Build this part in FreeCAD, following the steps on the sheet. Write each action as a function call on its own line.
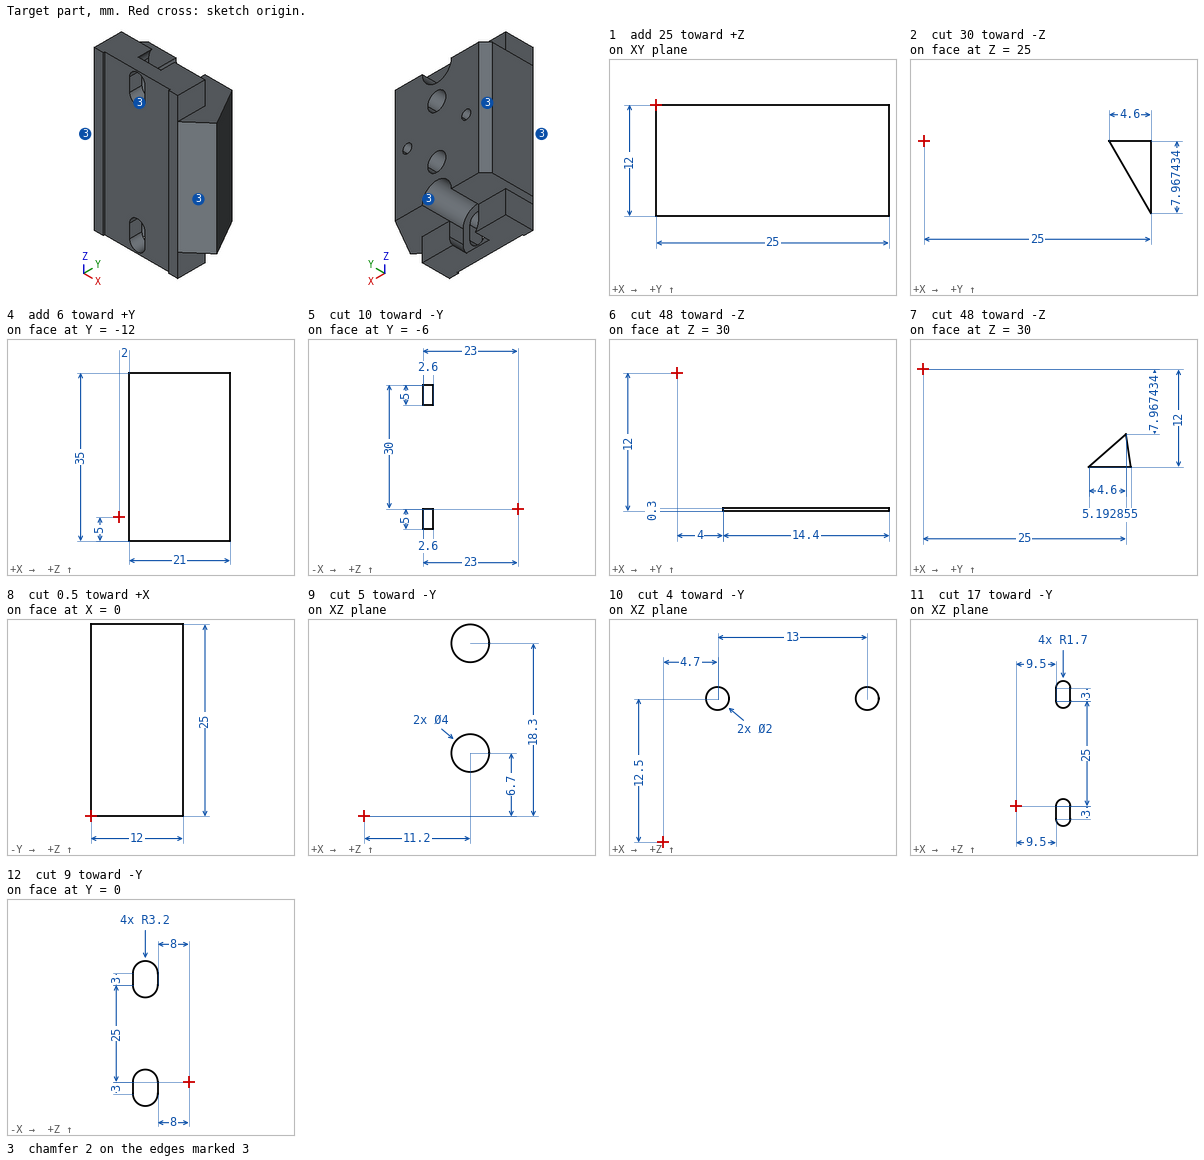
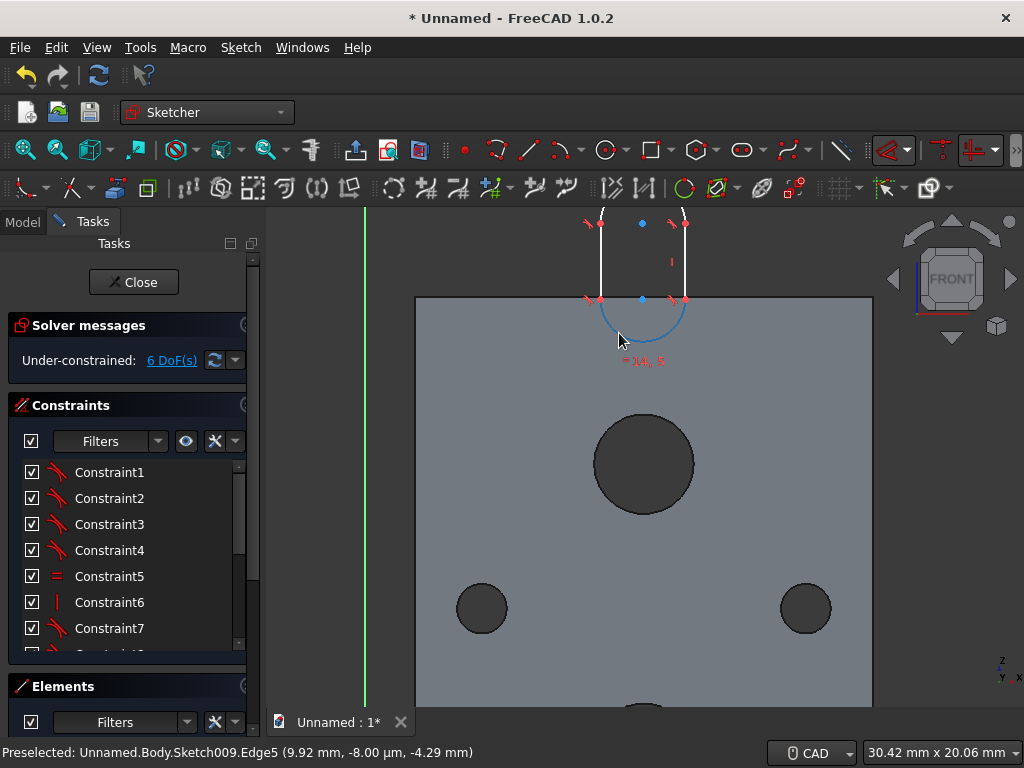
click(618, 334)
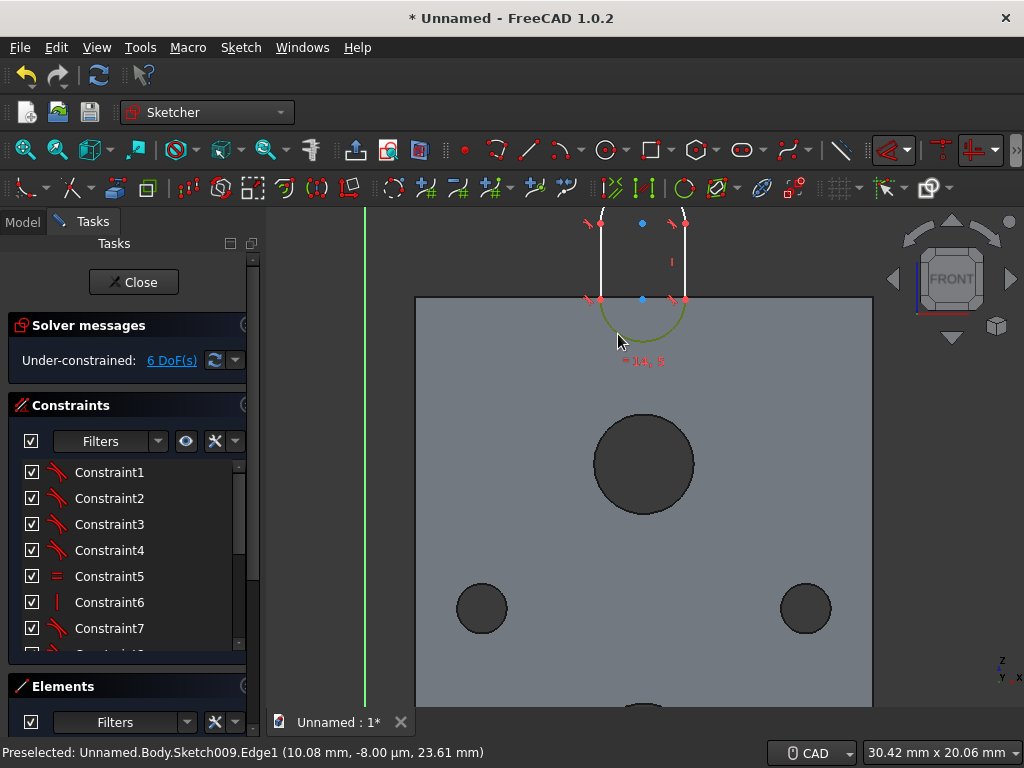
click(910, 150)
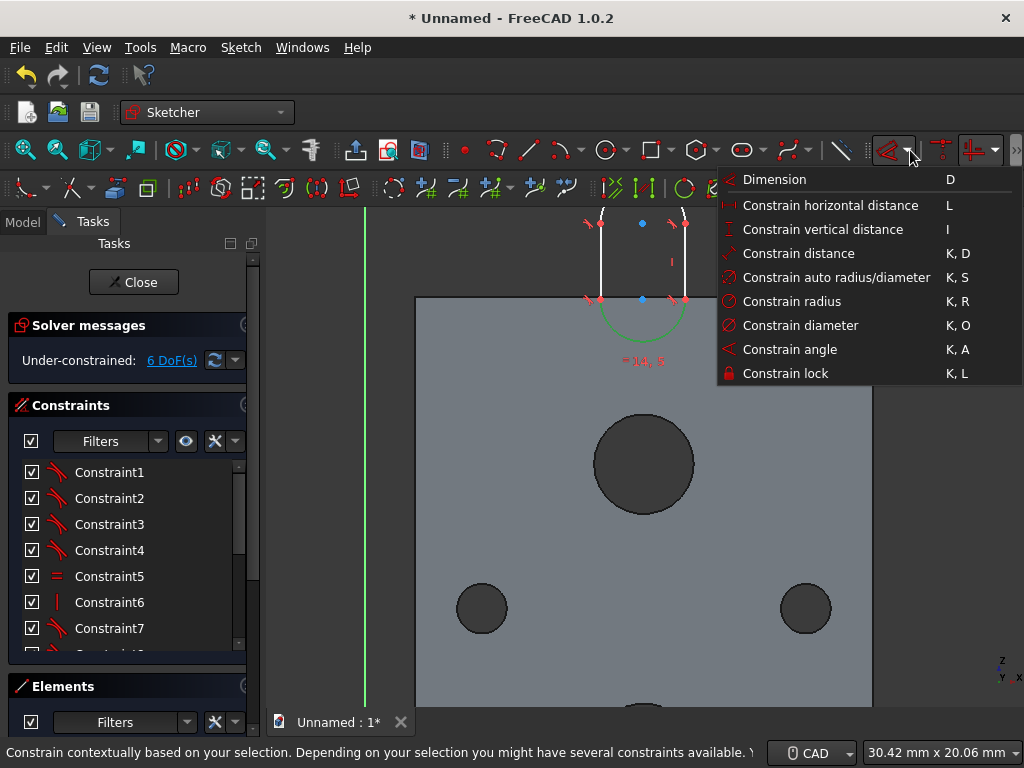
click(870, 301)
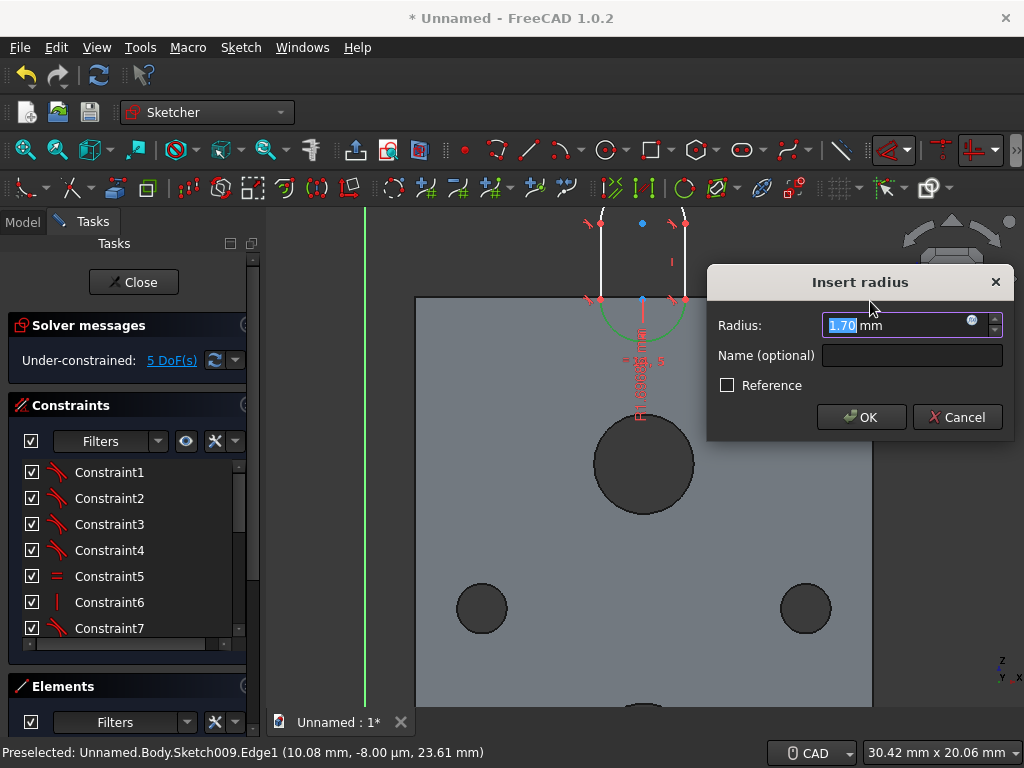
text(1.7)
key(Return)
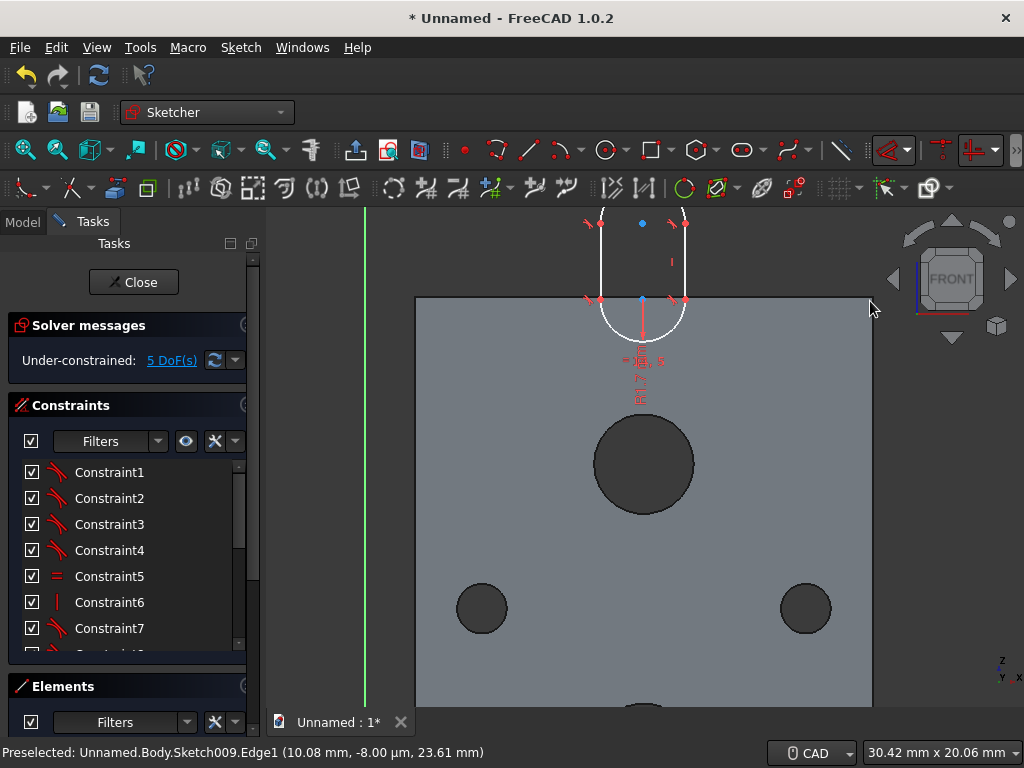
click(601, 277)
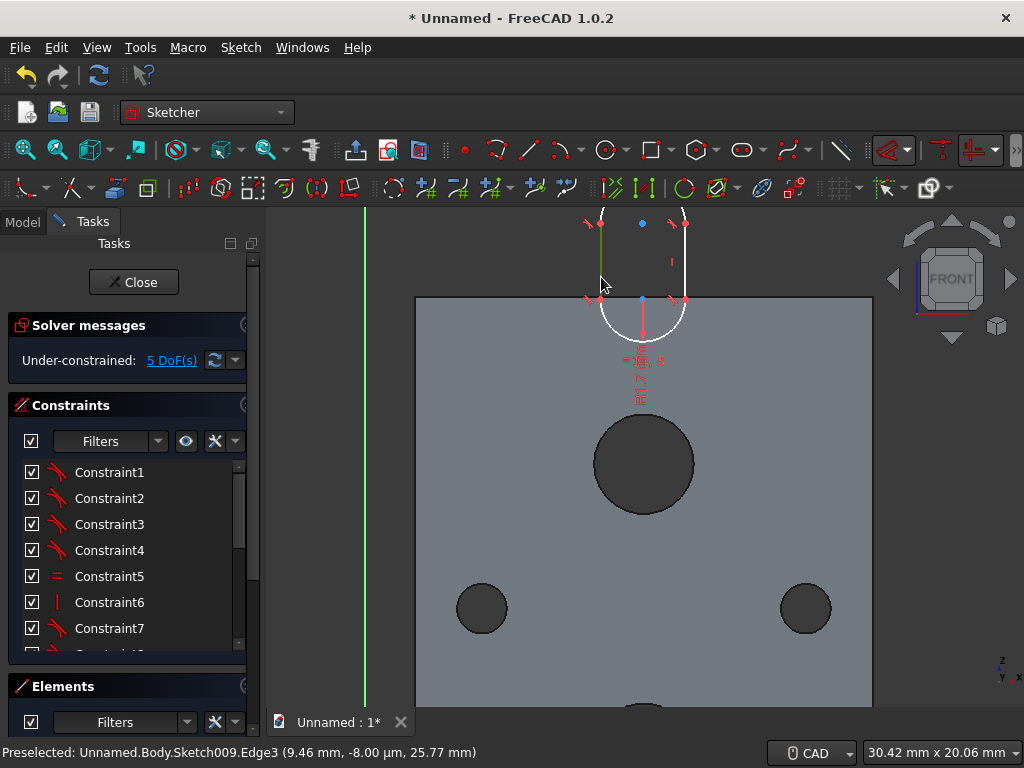
key(i)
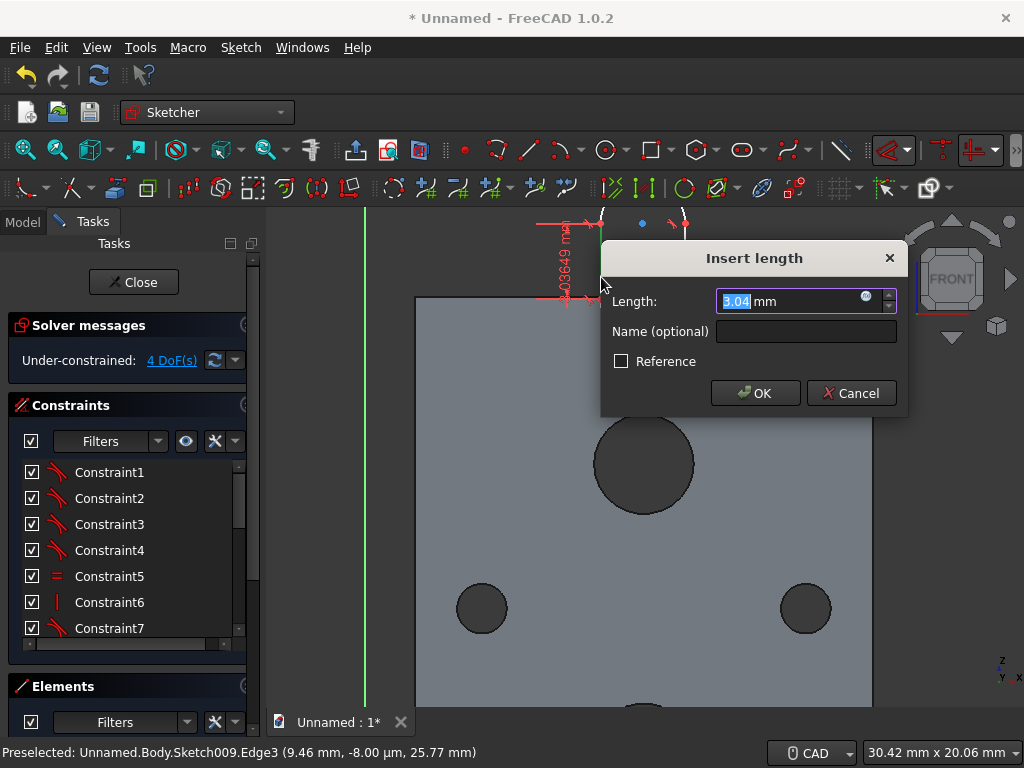
text(3)
key(Return)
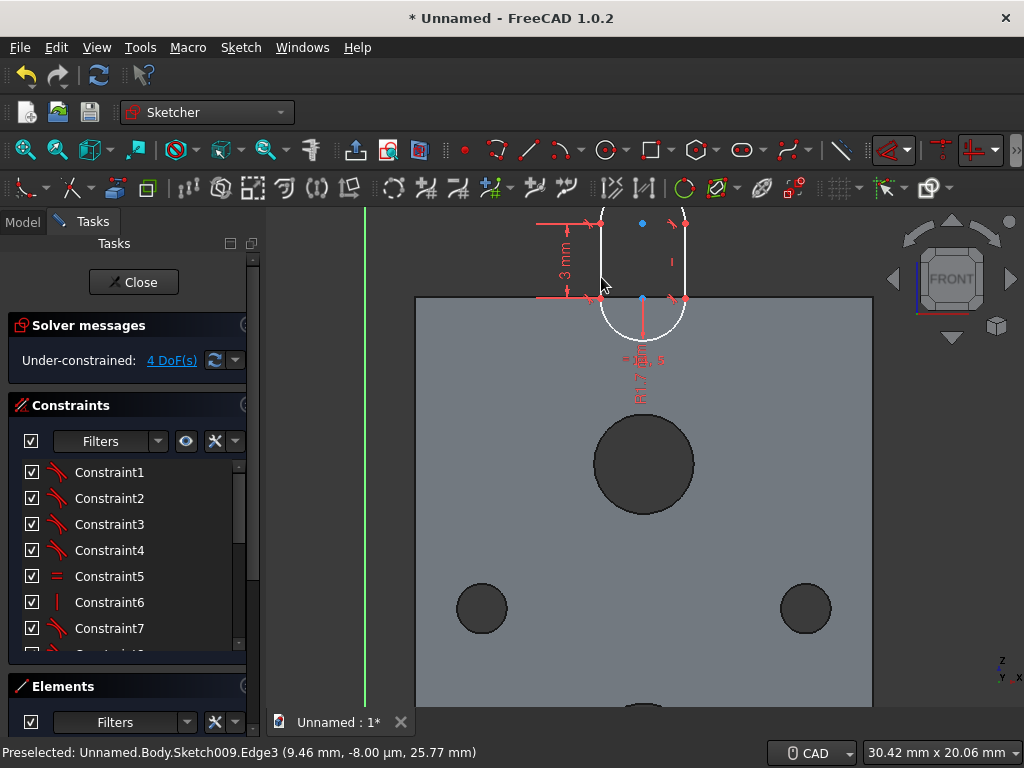
scroll(606, 369, down, 5)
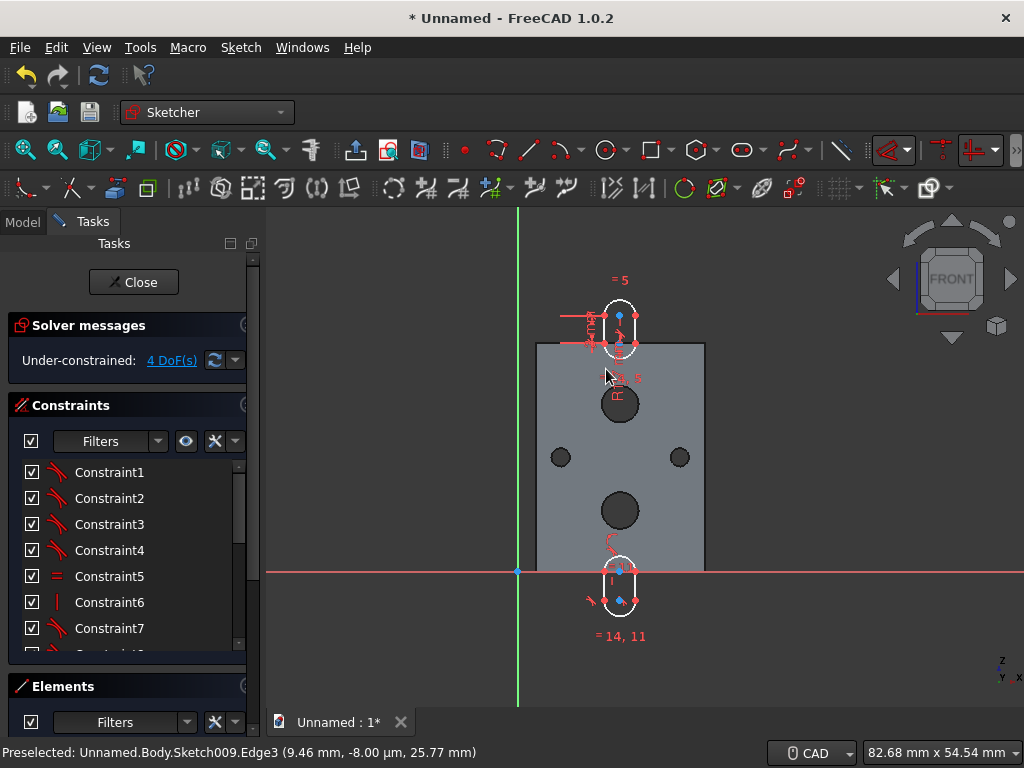
scroll(604, 592, up, 3)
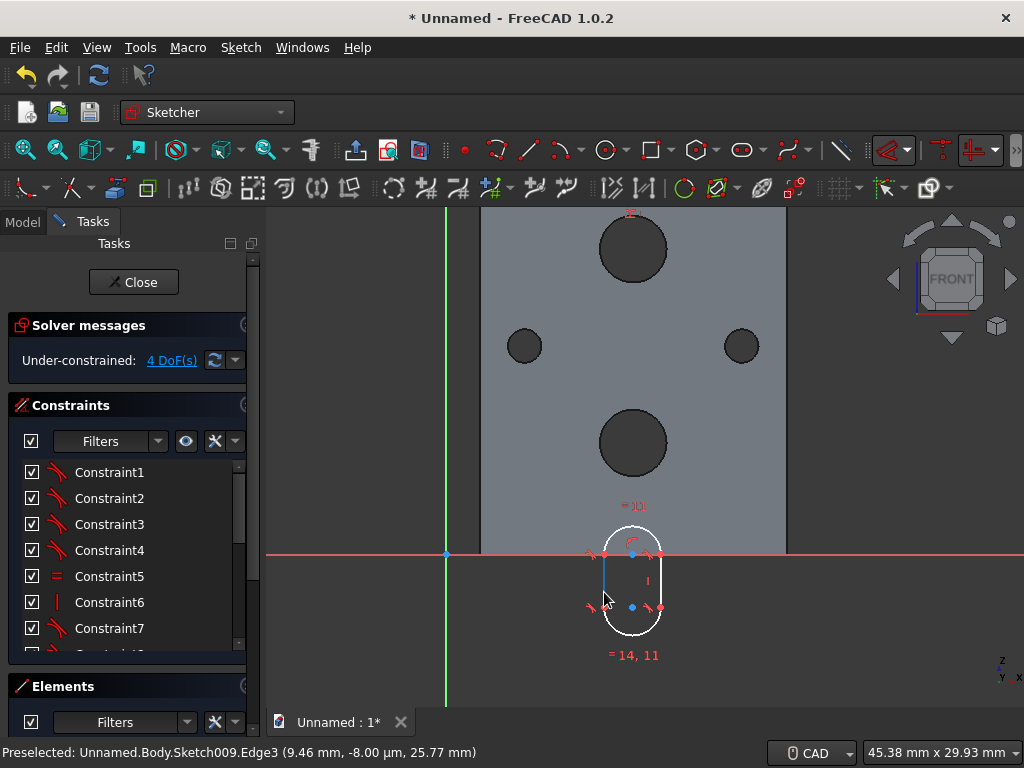
click(604, 591)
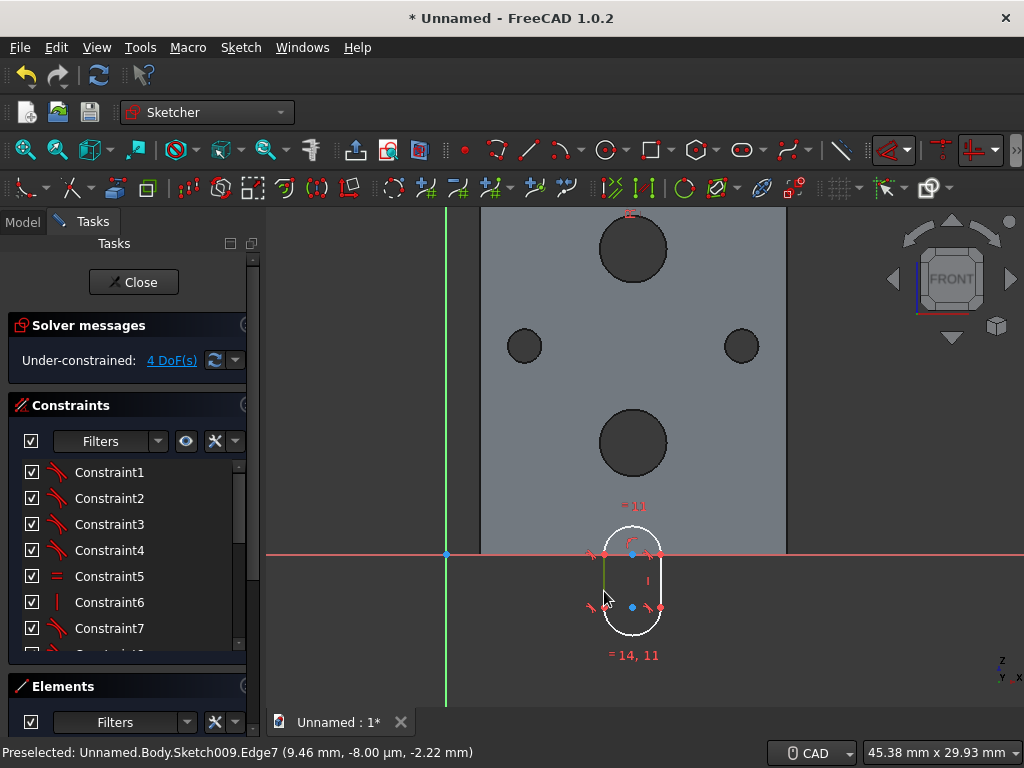
key(i)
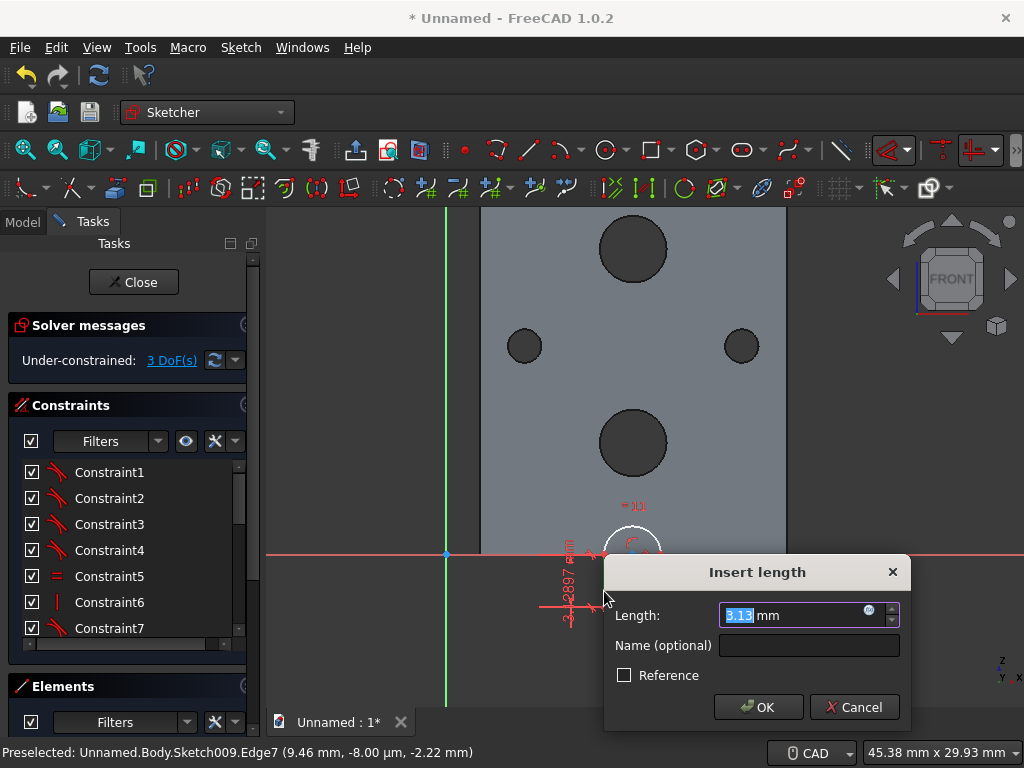
text(3)
key(Return)